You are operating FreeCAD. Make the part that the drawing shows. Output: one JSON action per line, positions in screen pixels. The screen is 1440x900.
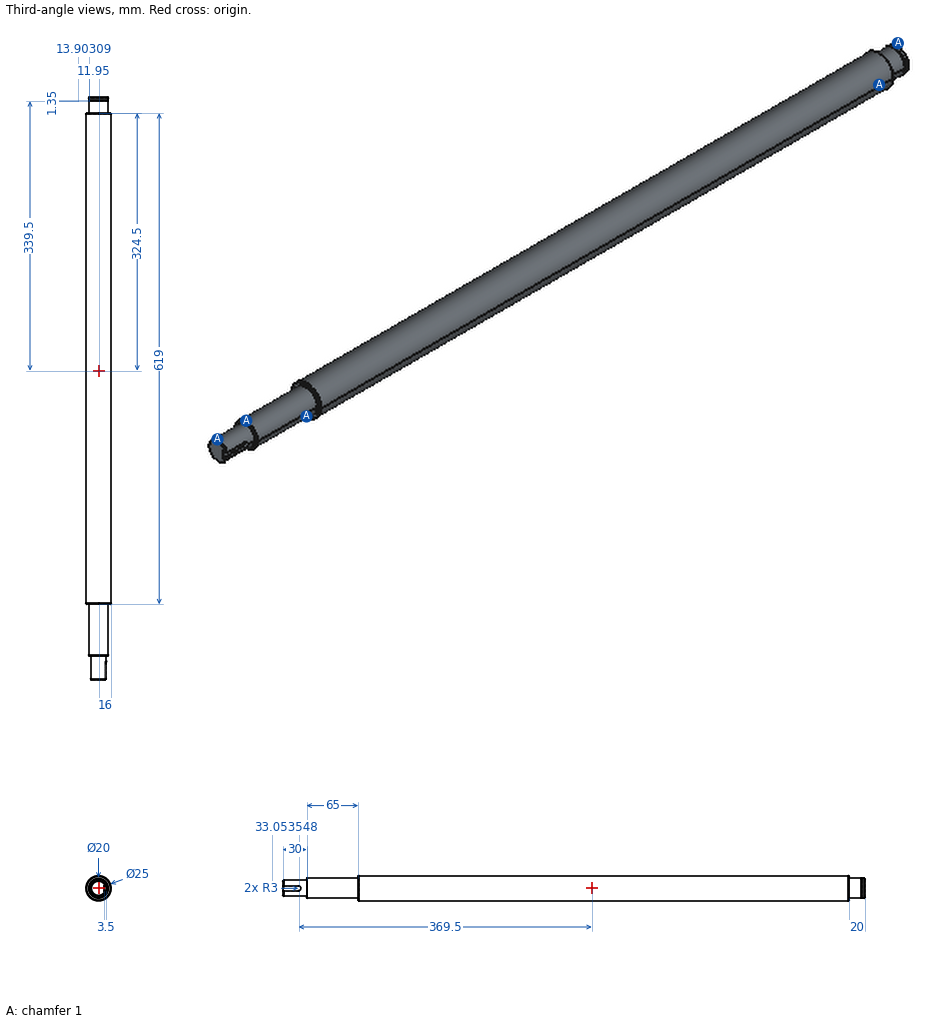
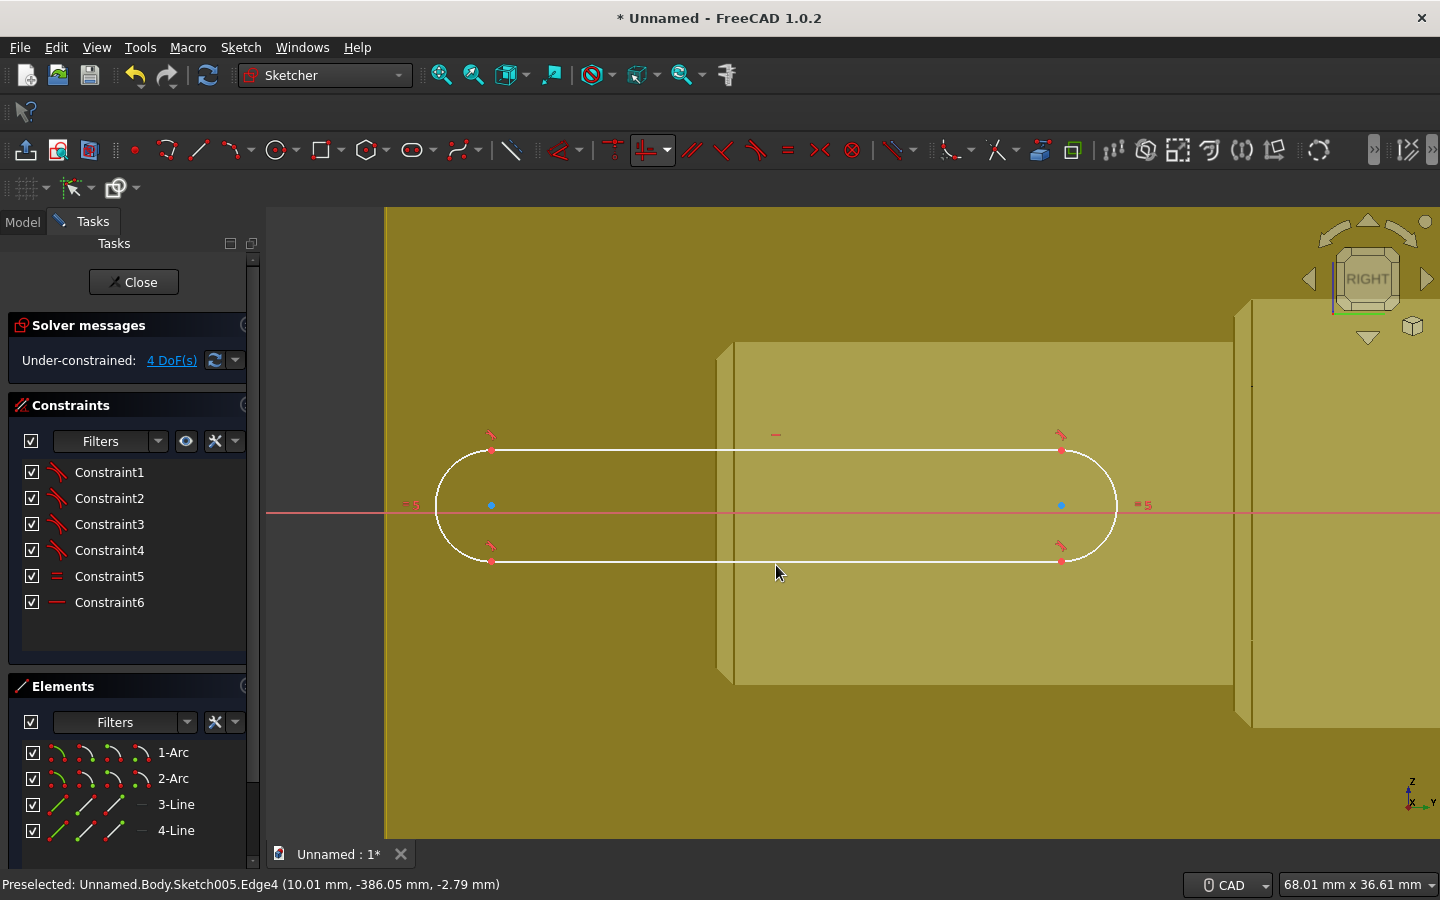
{"action": "left_click", "coordinate": [491, 506]}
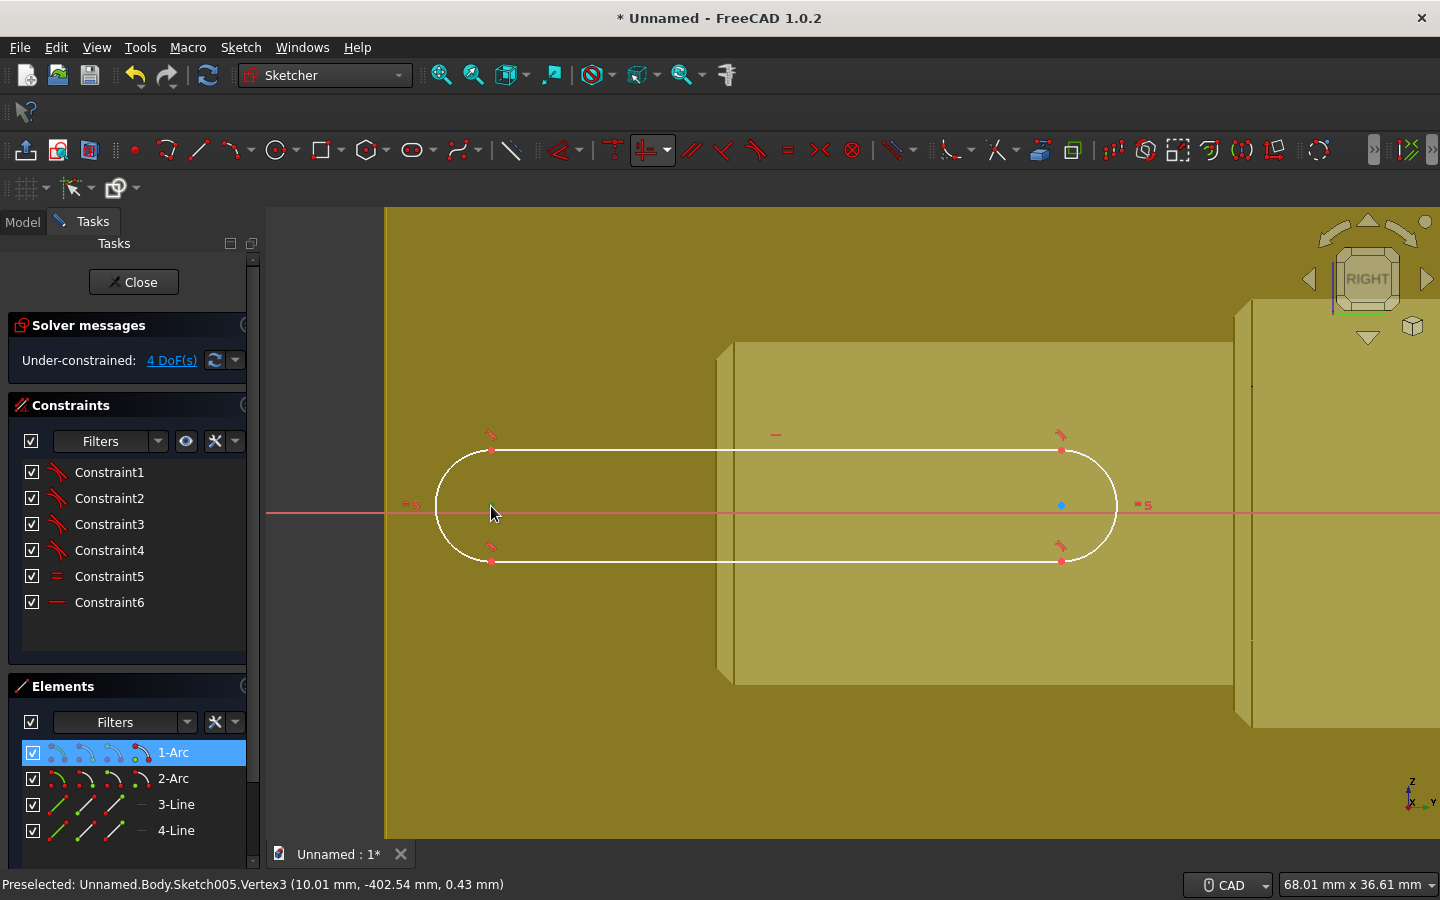
{"action": "left_click", "coordinate": [364, 513]}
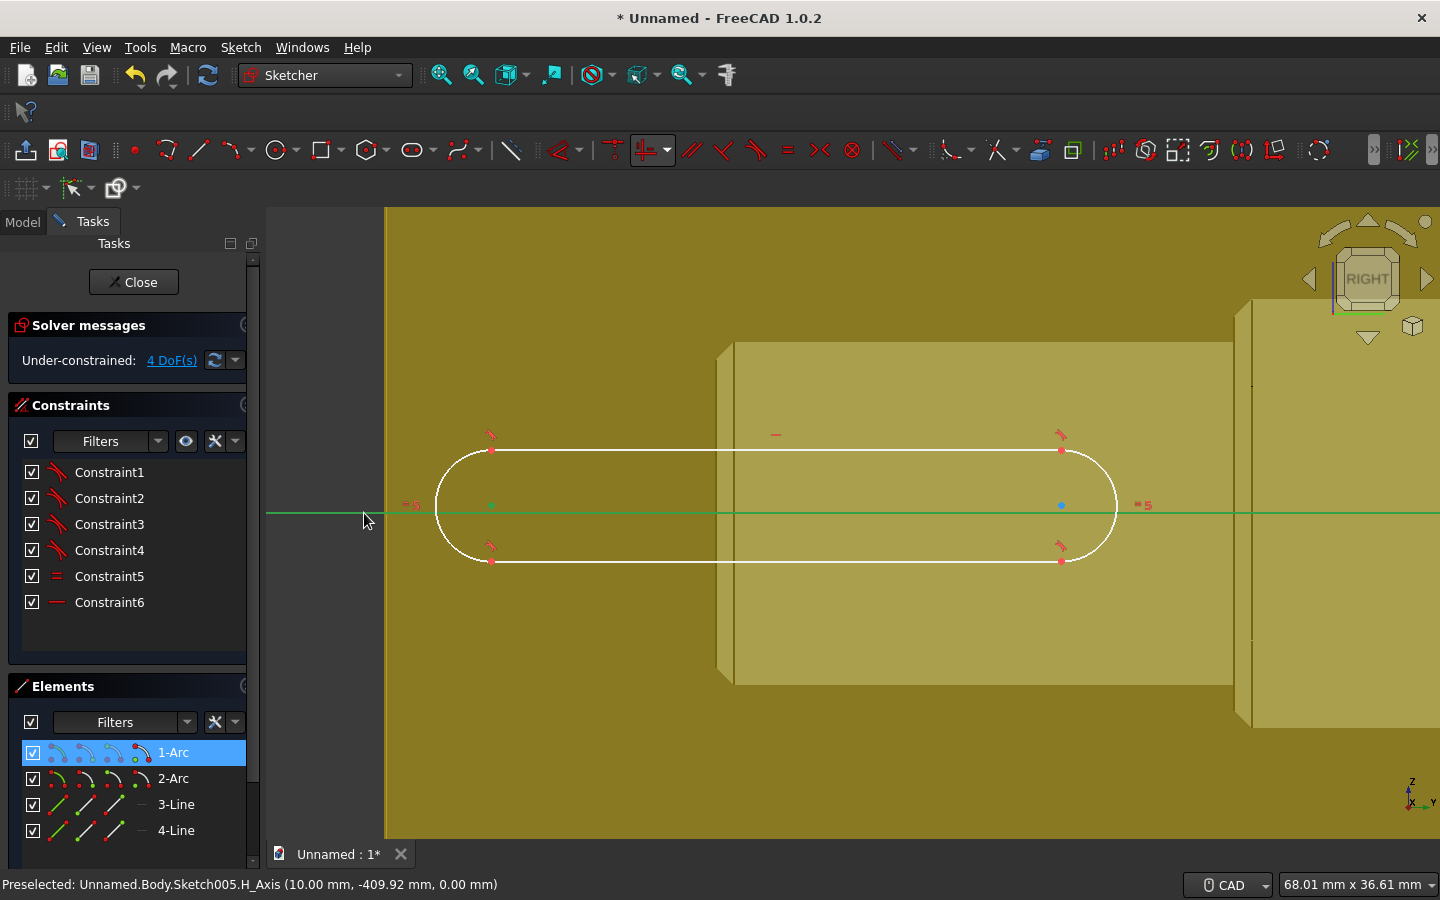
{"action": "left_click", "coordinate": [614, 150]}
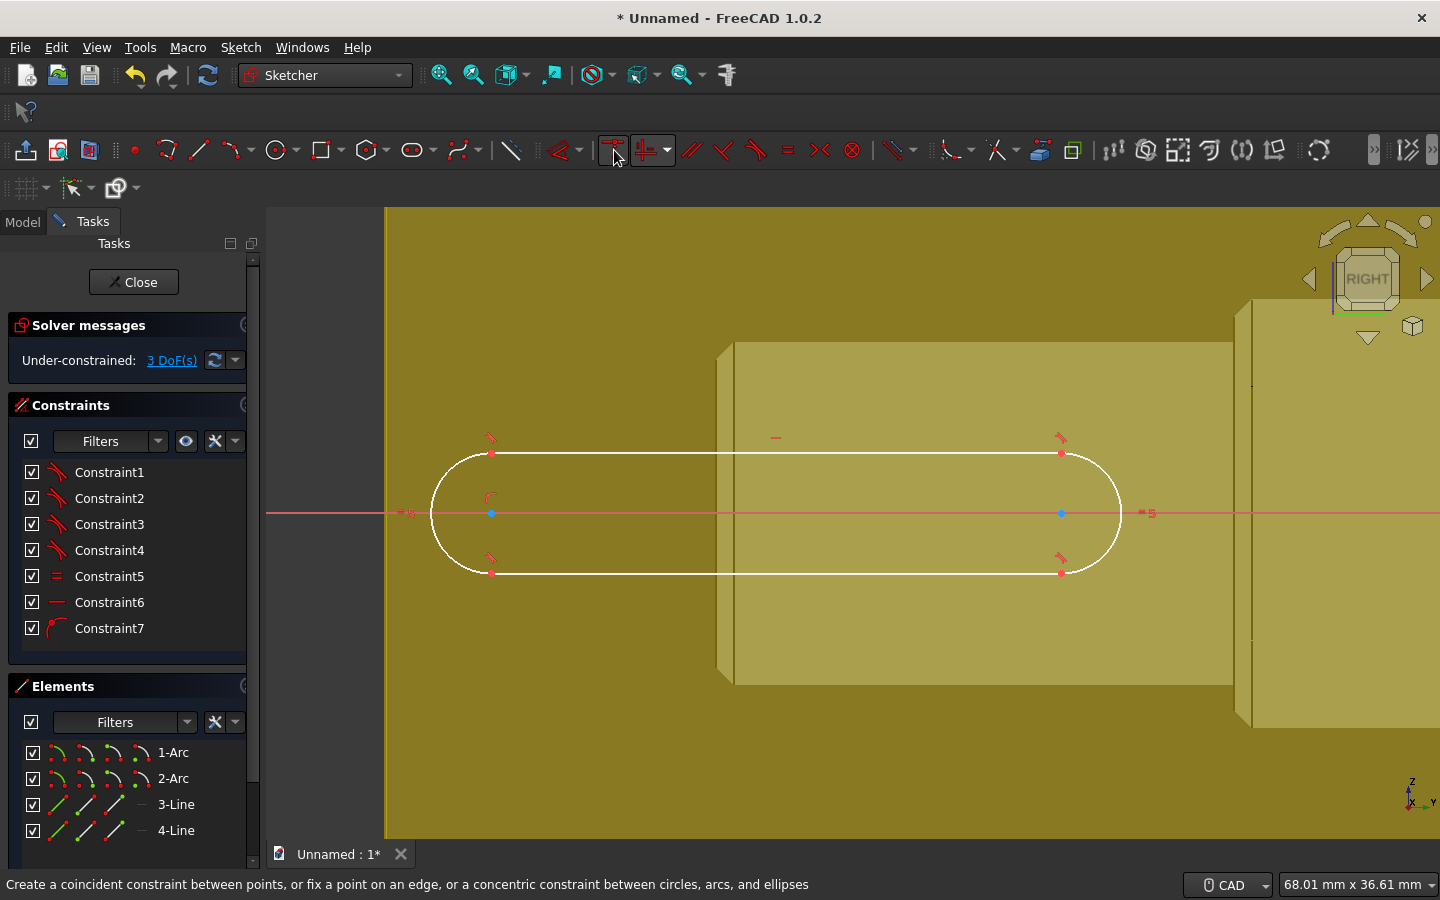
{"action": "left_click", "coordinate": [558, 150]}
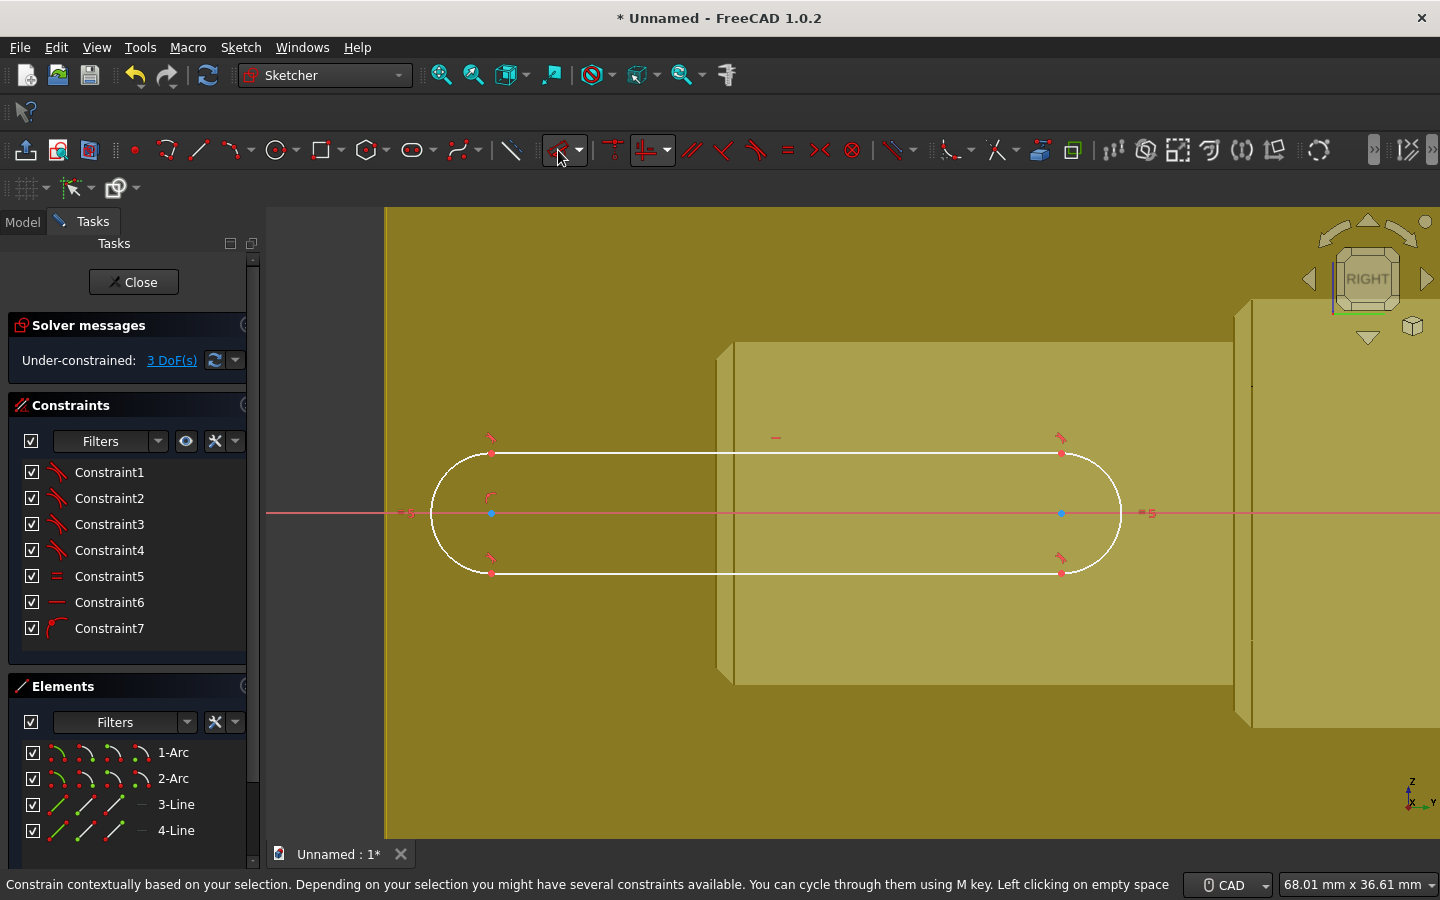
{"action": "left_click", "coordinate": [443, 478]}
{"action": "left_click", "coordinate": [417, 459]}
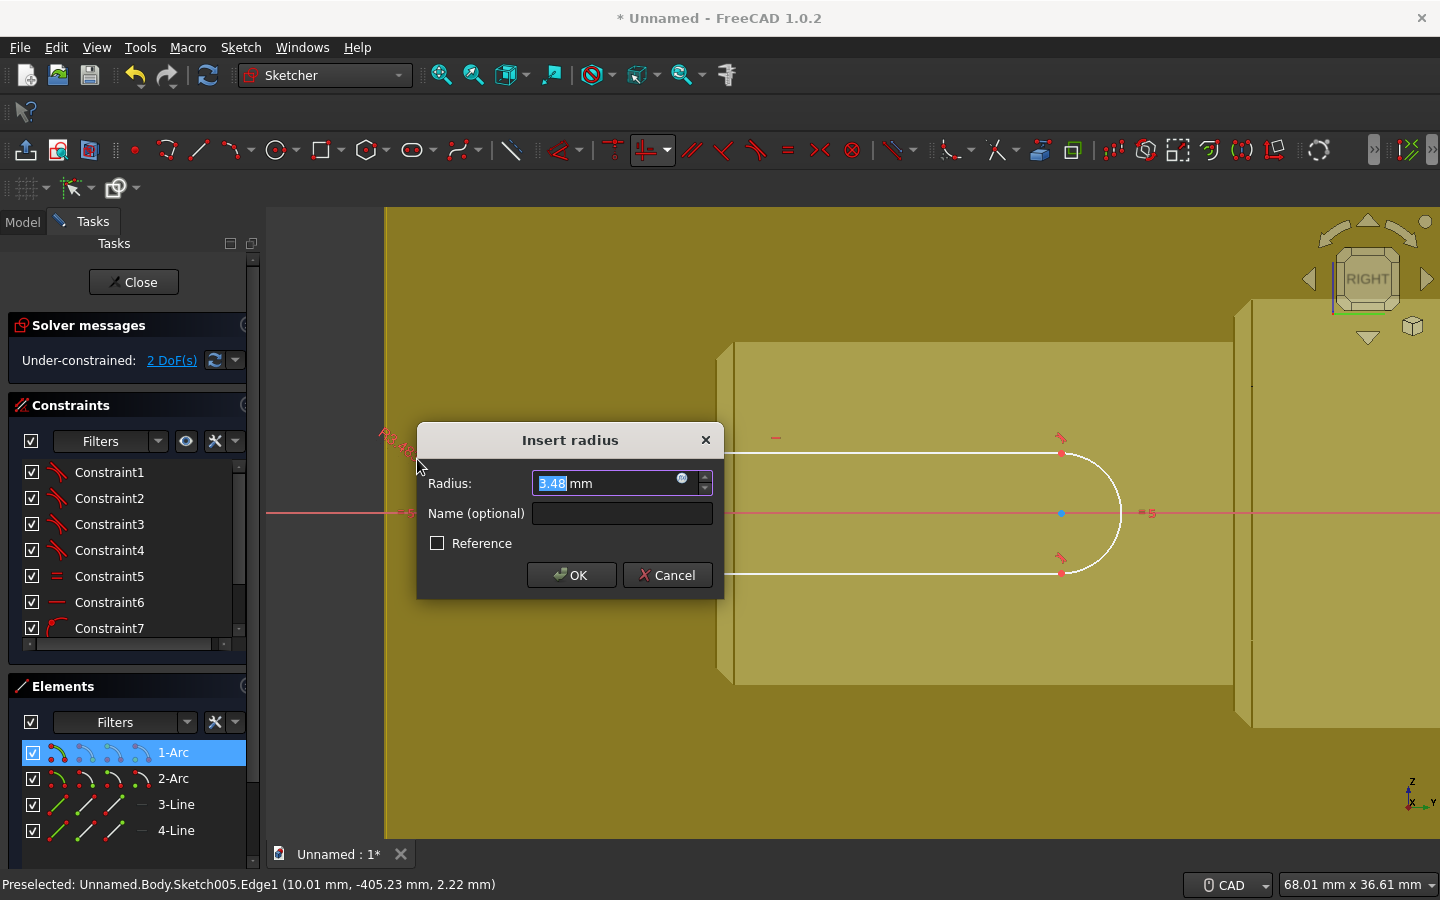
{"action": "type", "text": "3"}
{"action": "key", "text": "Return"}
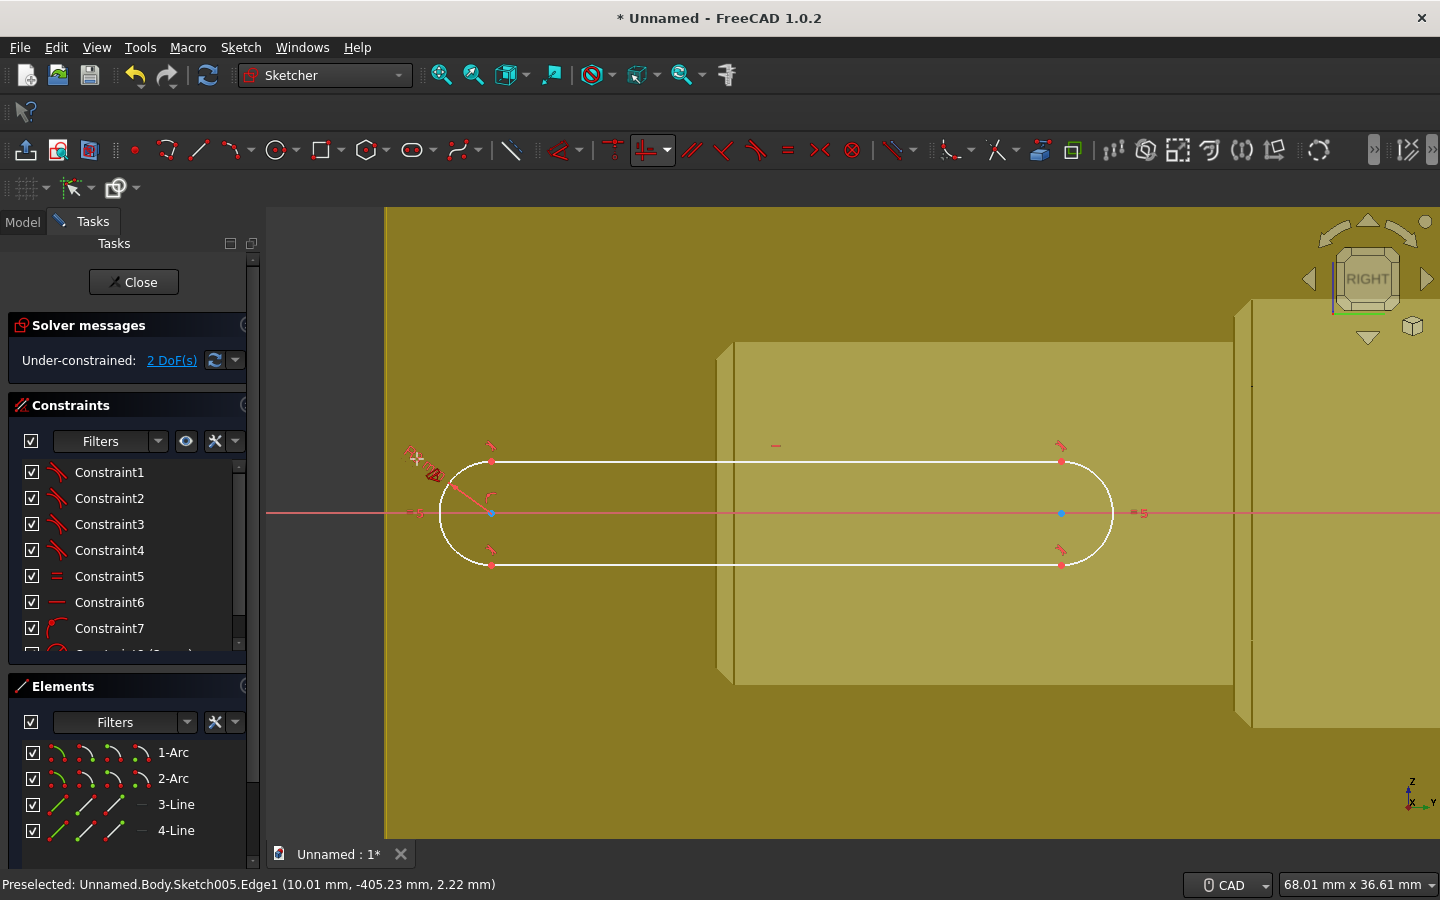
{"action": "left_click", "coordinate": [1061, 565]}
{"action": "left_click", "coordinate": [1168, 599]}